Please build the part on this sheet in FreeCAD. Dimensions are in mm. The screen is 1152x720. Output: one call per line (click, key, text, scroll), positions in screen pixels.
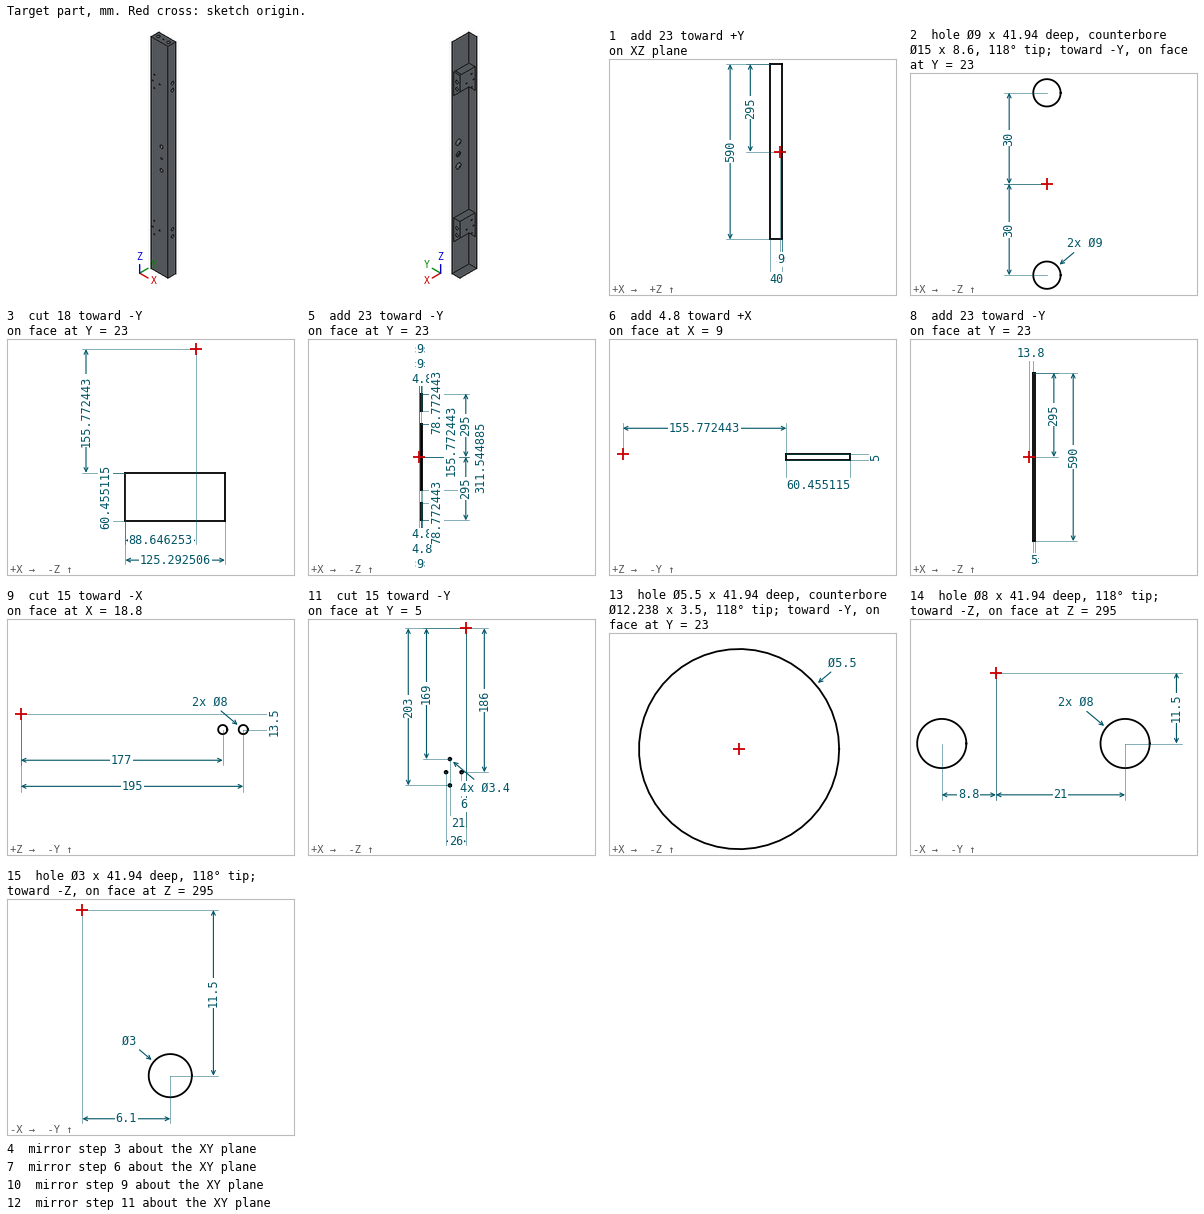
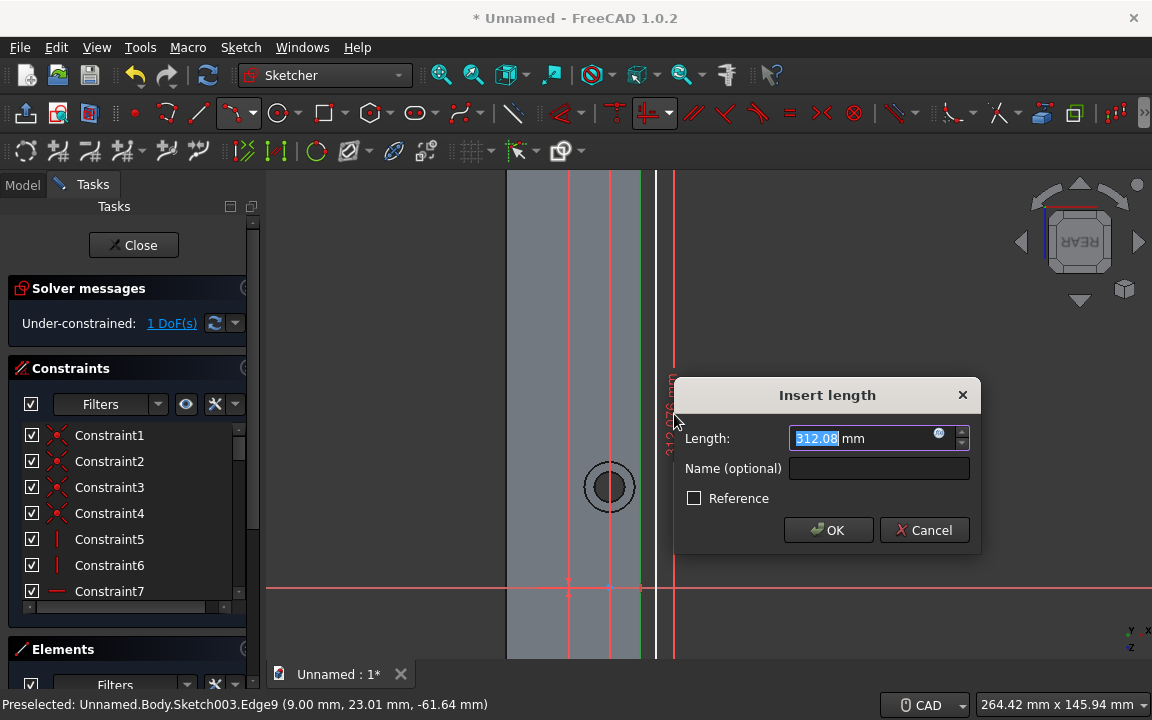
text(311.544885)
key(Return)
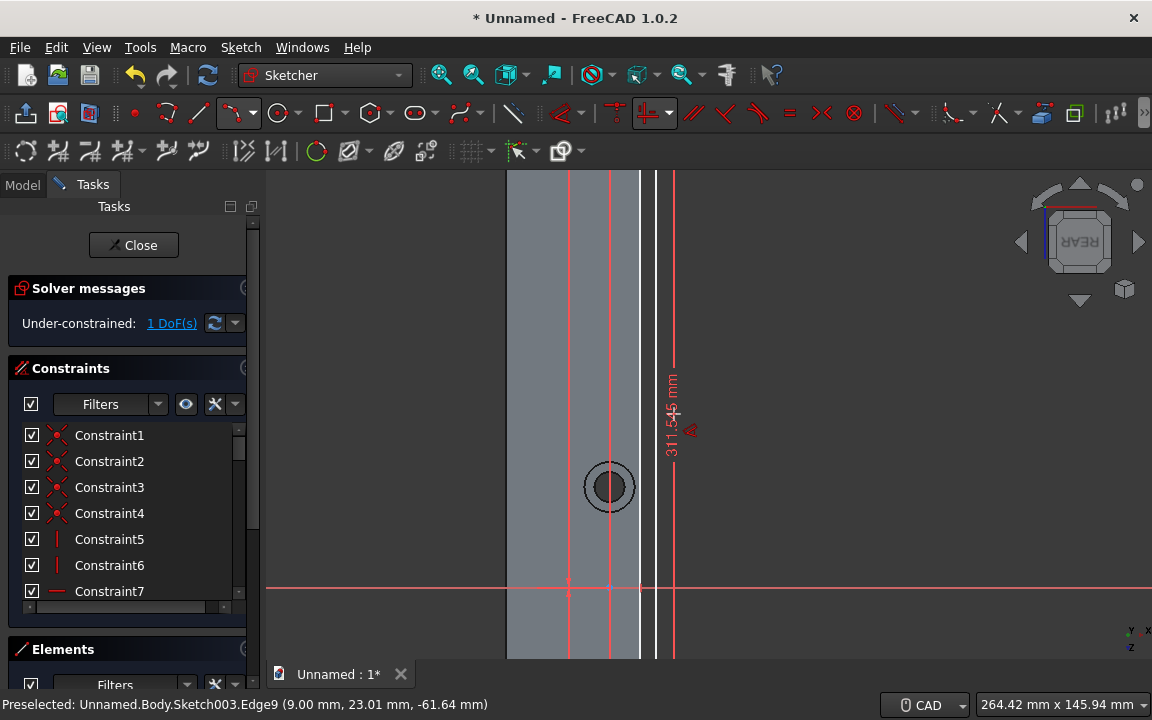
scroll(642, 380, down, 9)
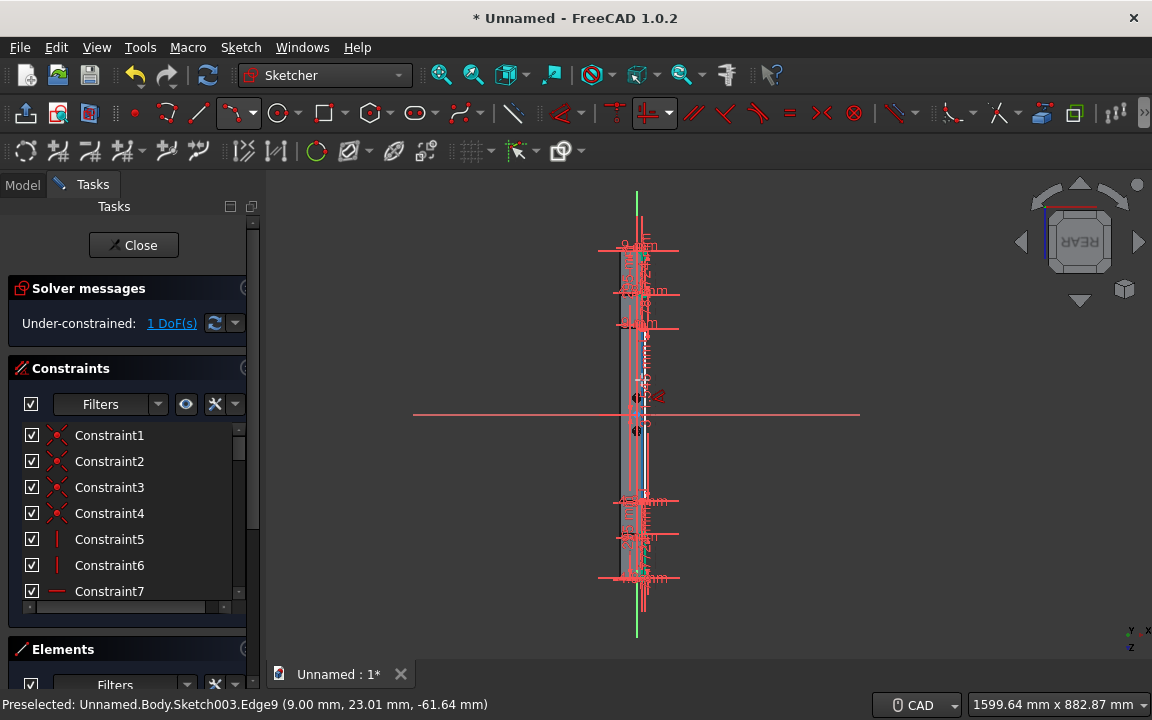
scroll(642, 329, up, 8)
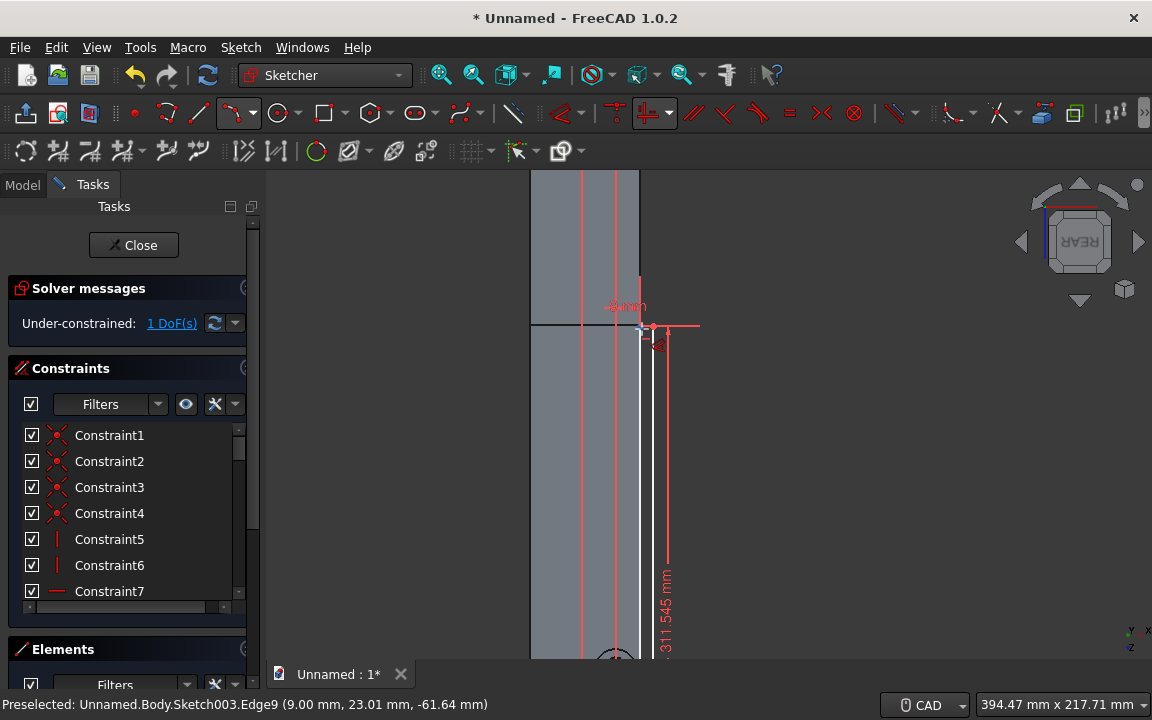
click(640, 326)
click(582, 479)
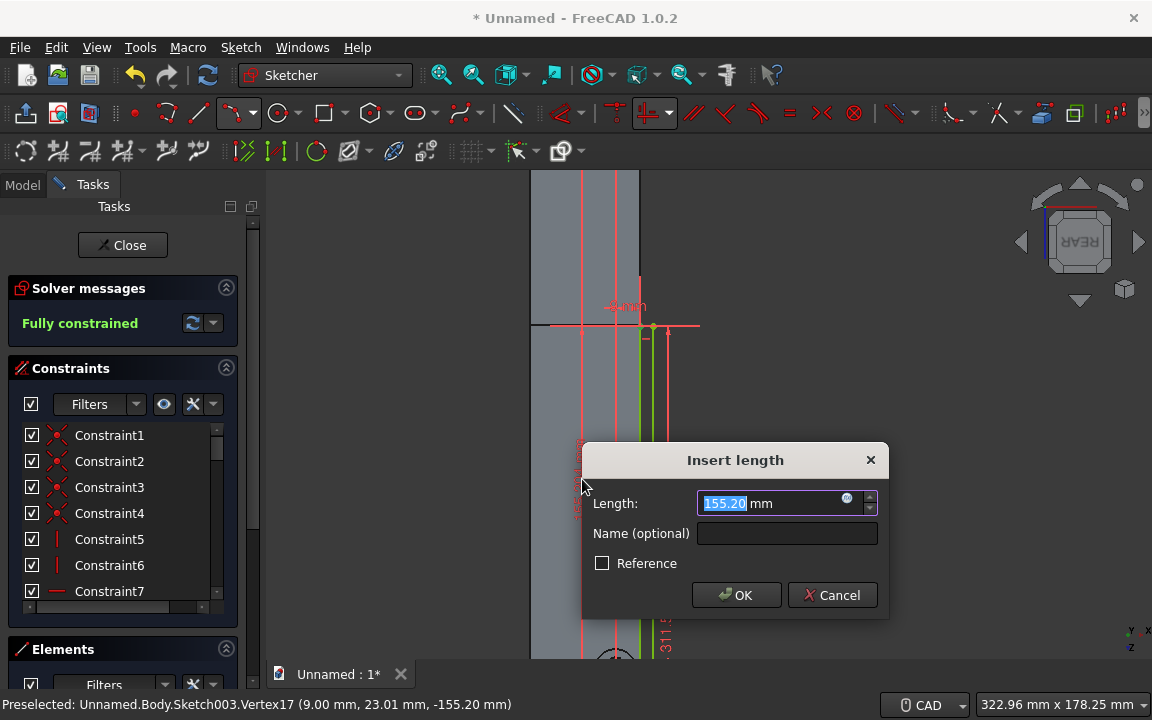
text(155.772443)
key(Return)
key(Escape)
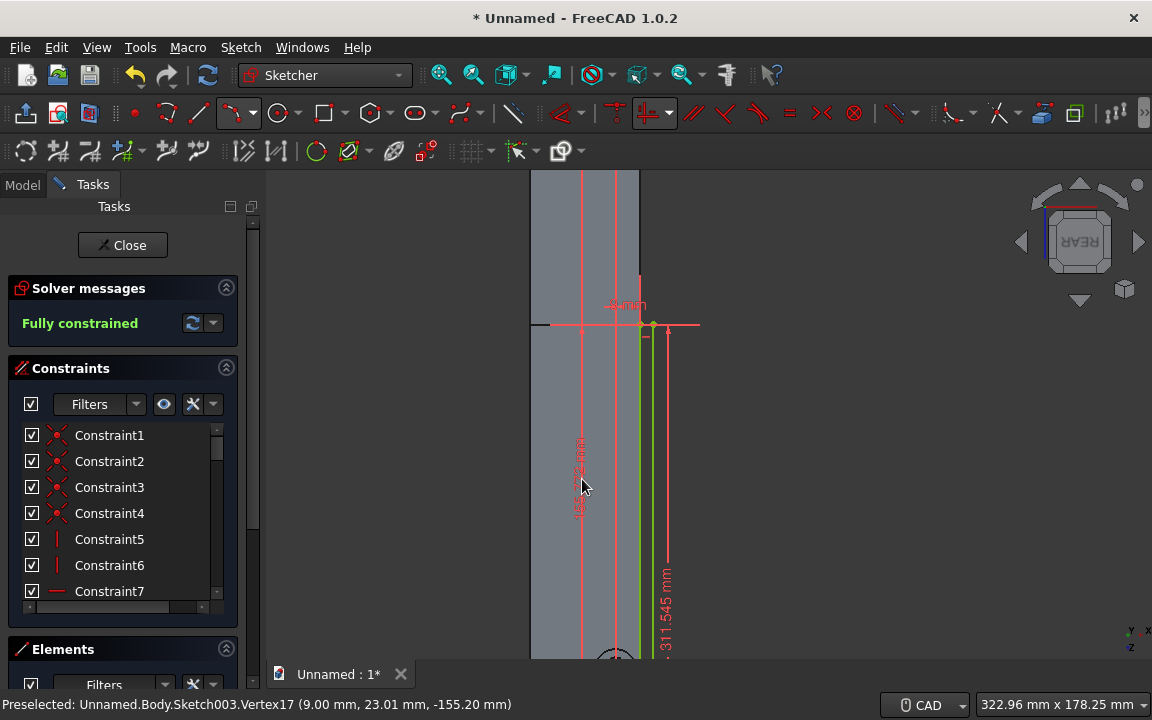
click(123, 245)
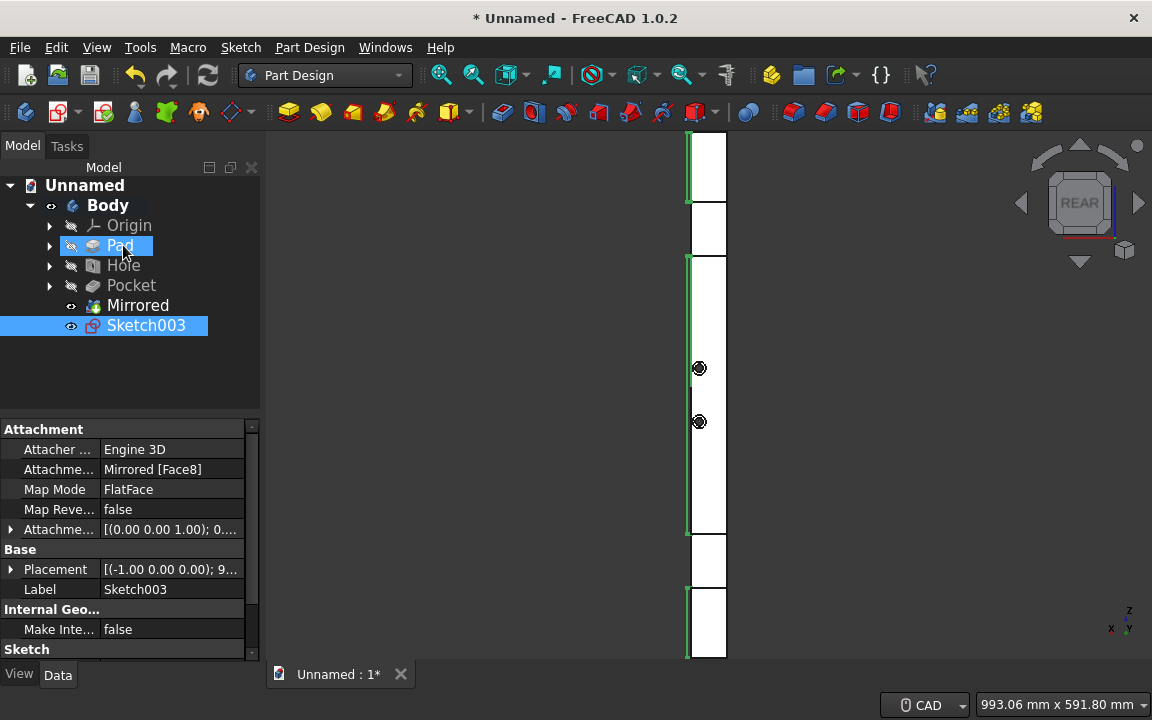
click(290, 112)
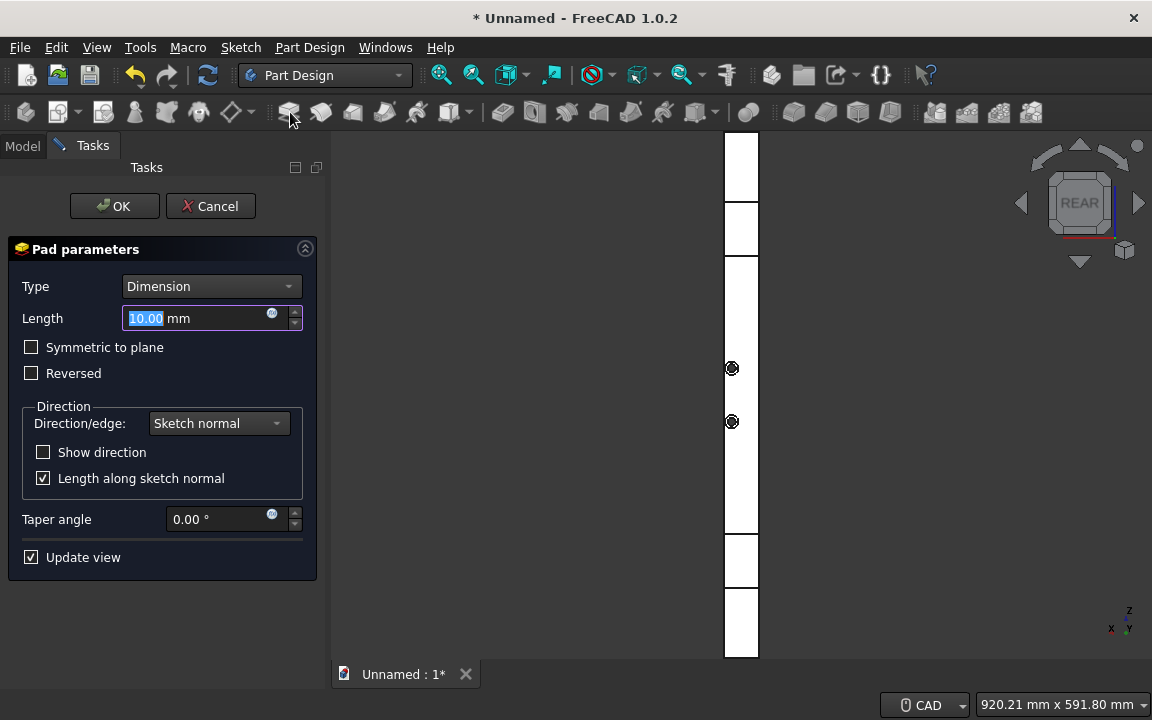
text(23)
key(Tab)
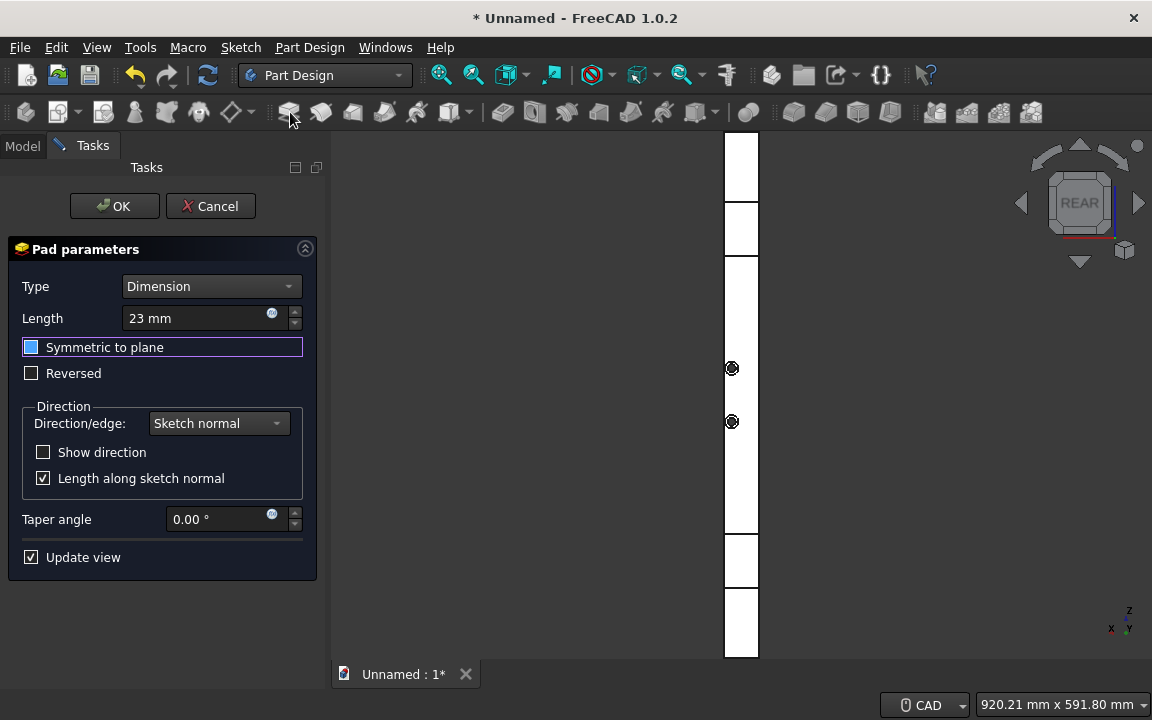
click(30, 373)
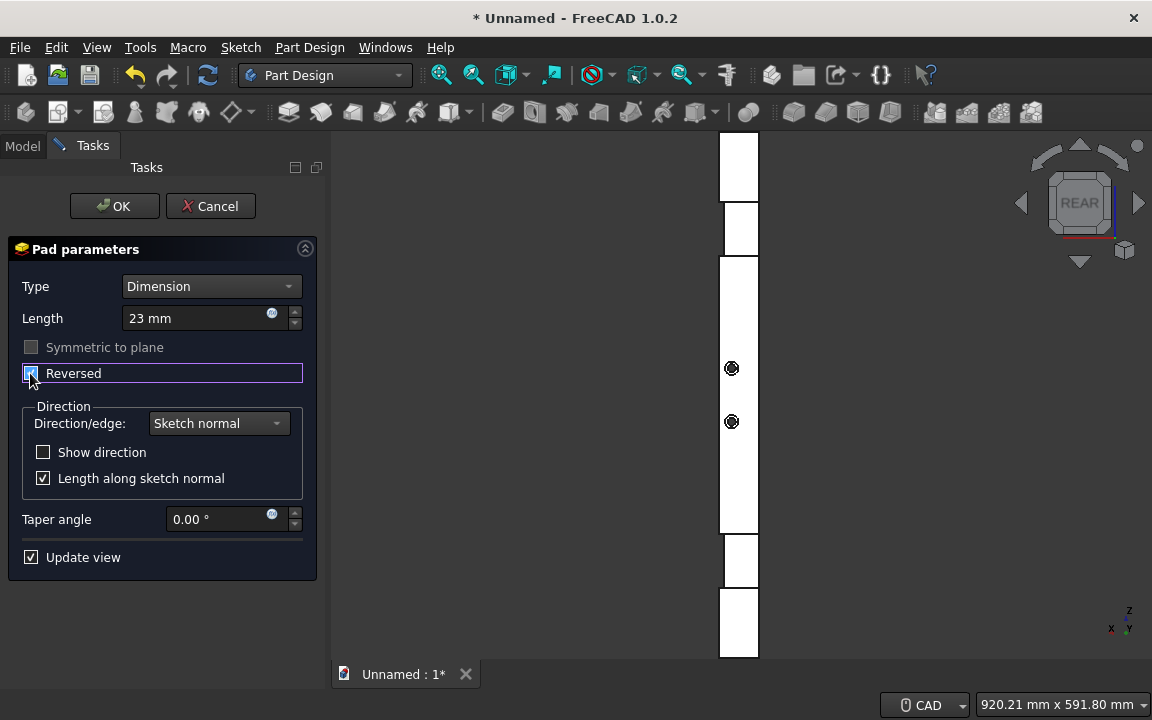
click(115, 206)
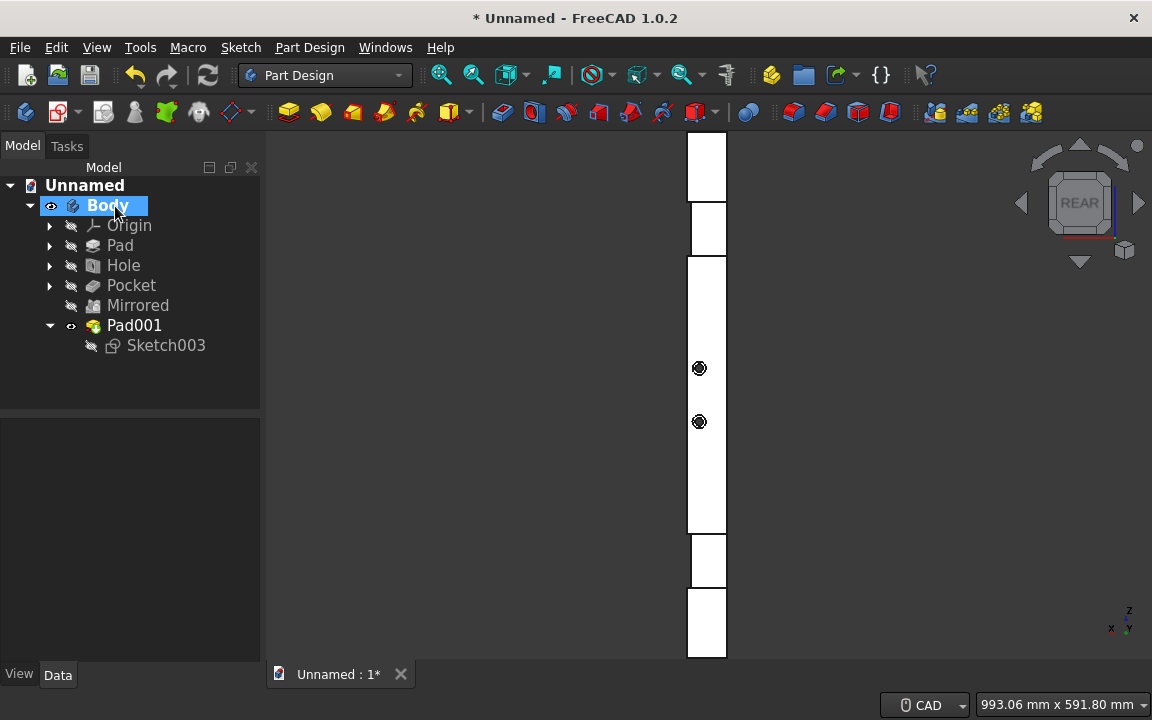
key(0)